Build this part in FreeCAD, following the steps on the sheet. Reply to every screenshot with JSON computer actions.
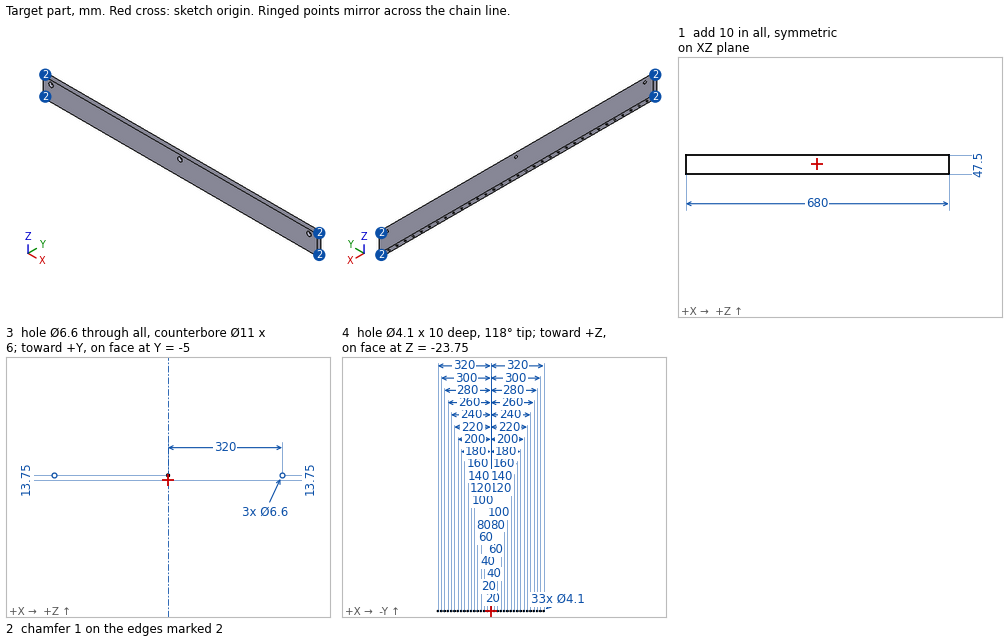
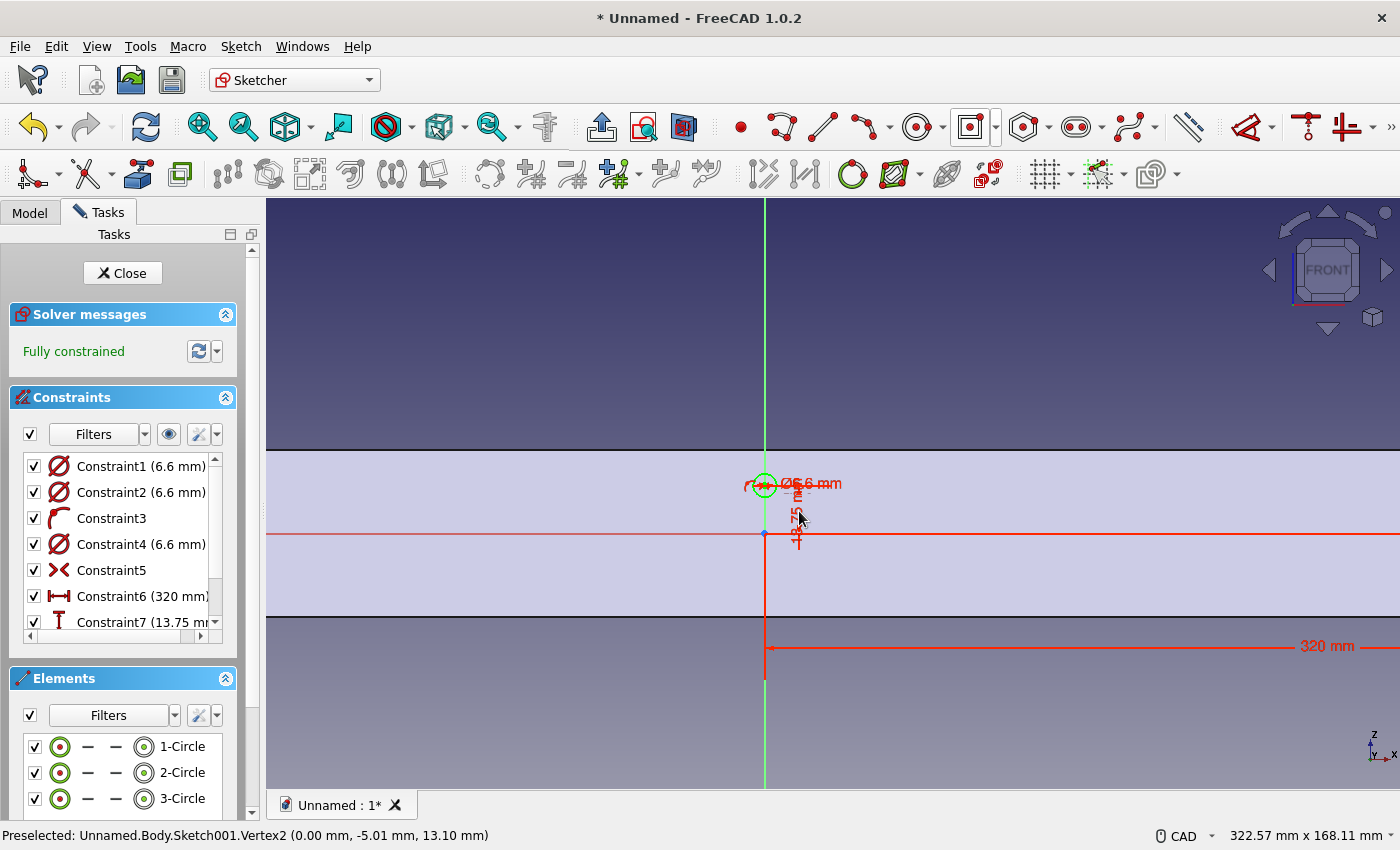
{"action": "left_click", "coordinate": [123, 273]}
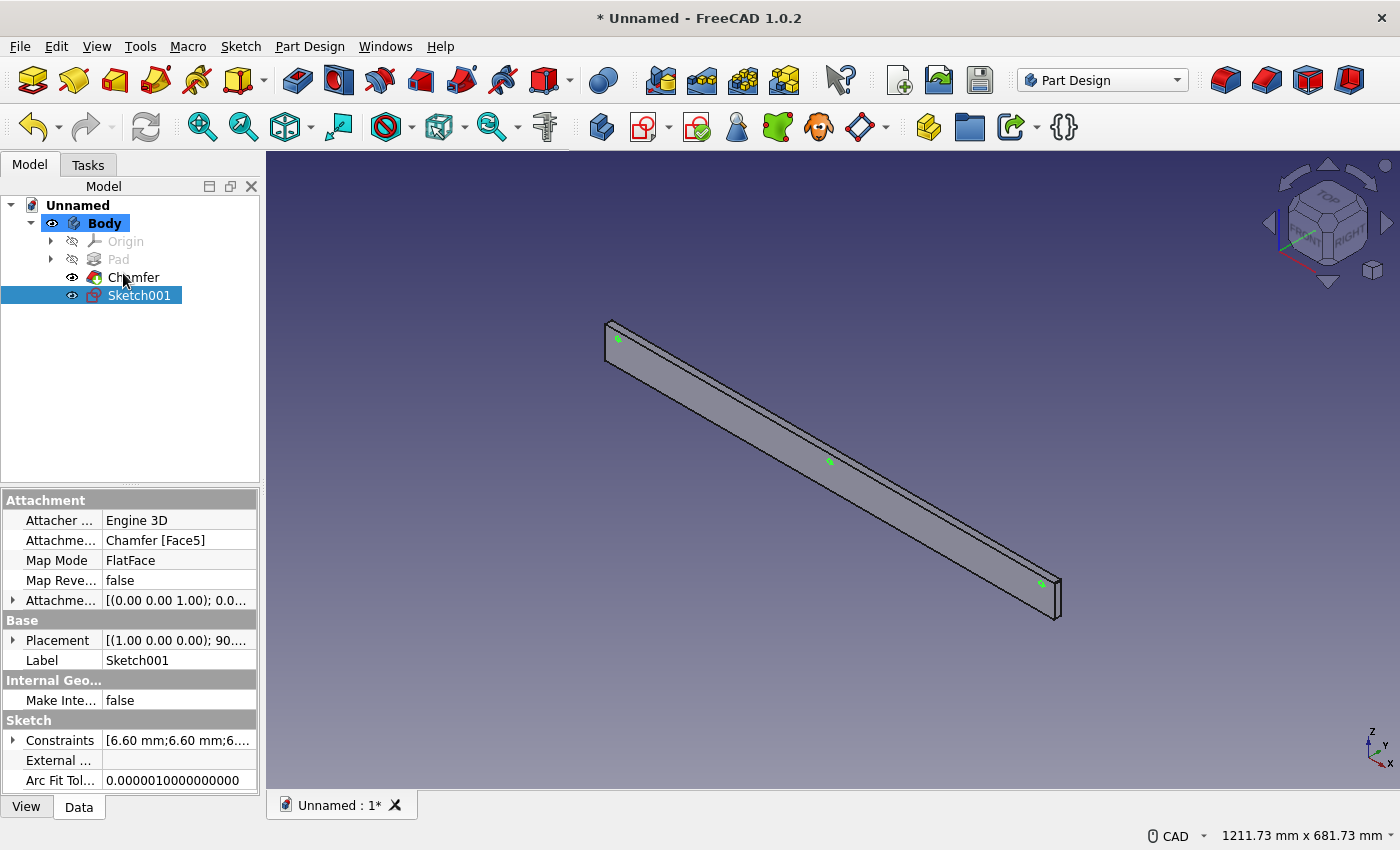
{"action": "left_click", "coordinate": [339, 80]}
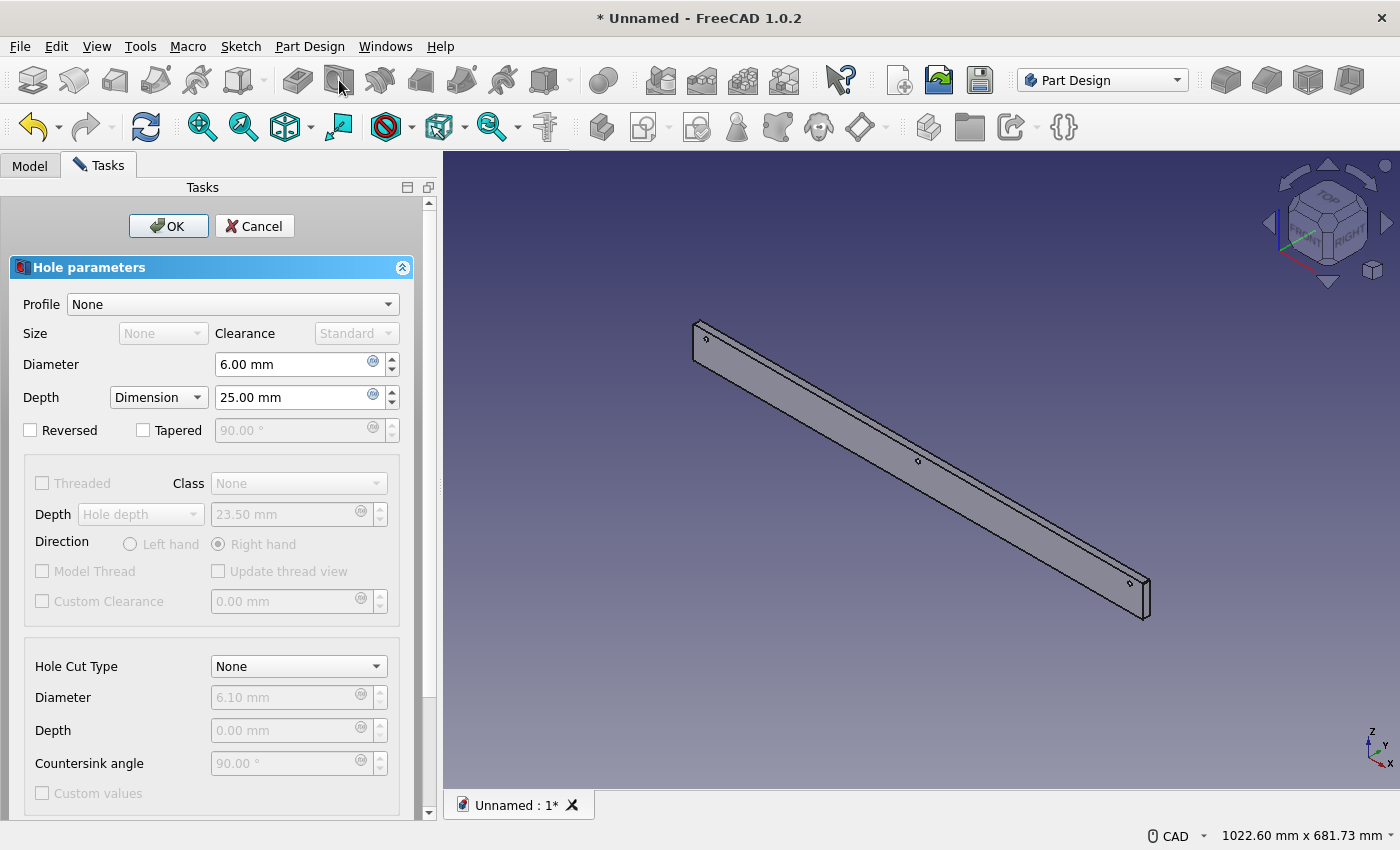
{"action": "triple_click", "coordinate": [300, 364]}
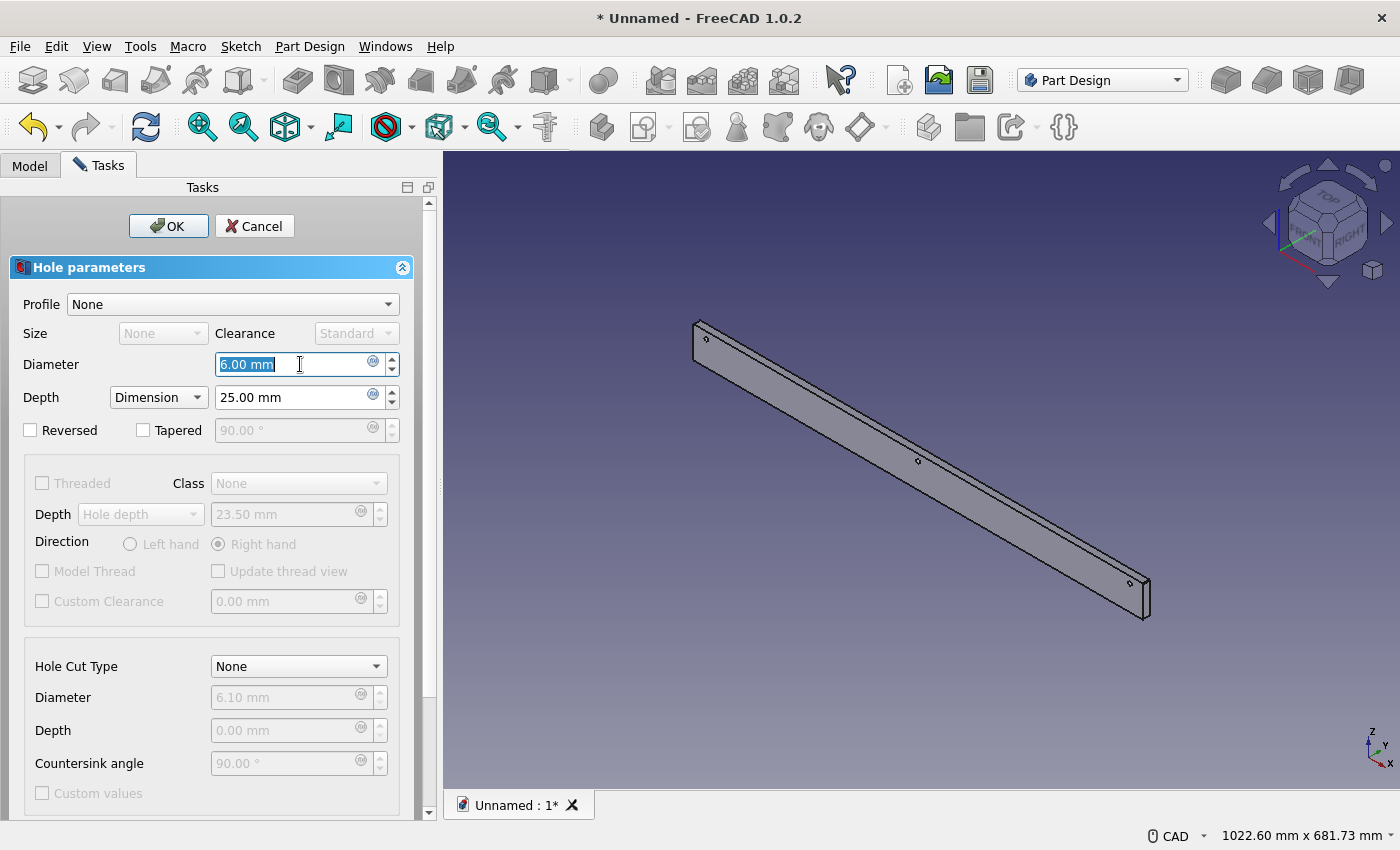
{"action": "type", "text": "6.6"}
{"action": "key", "text": "Tab"}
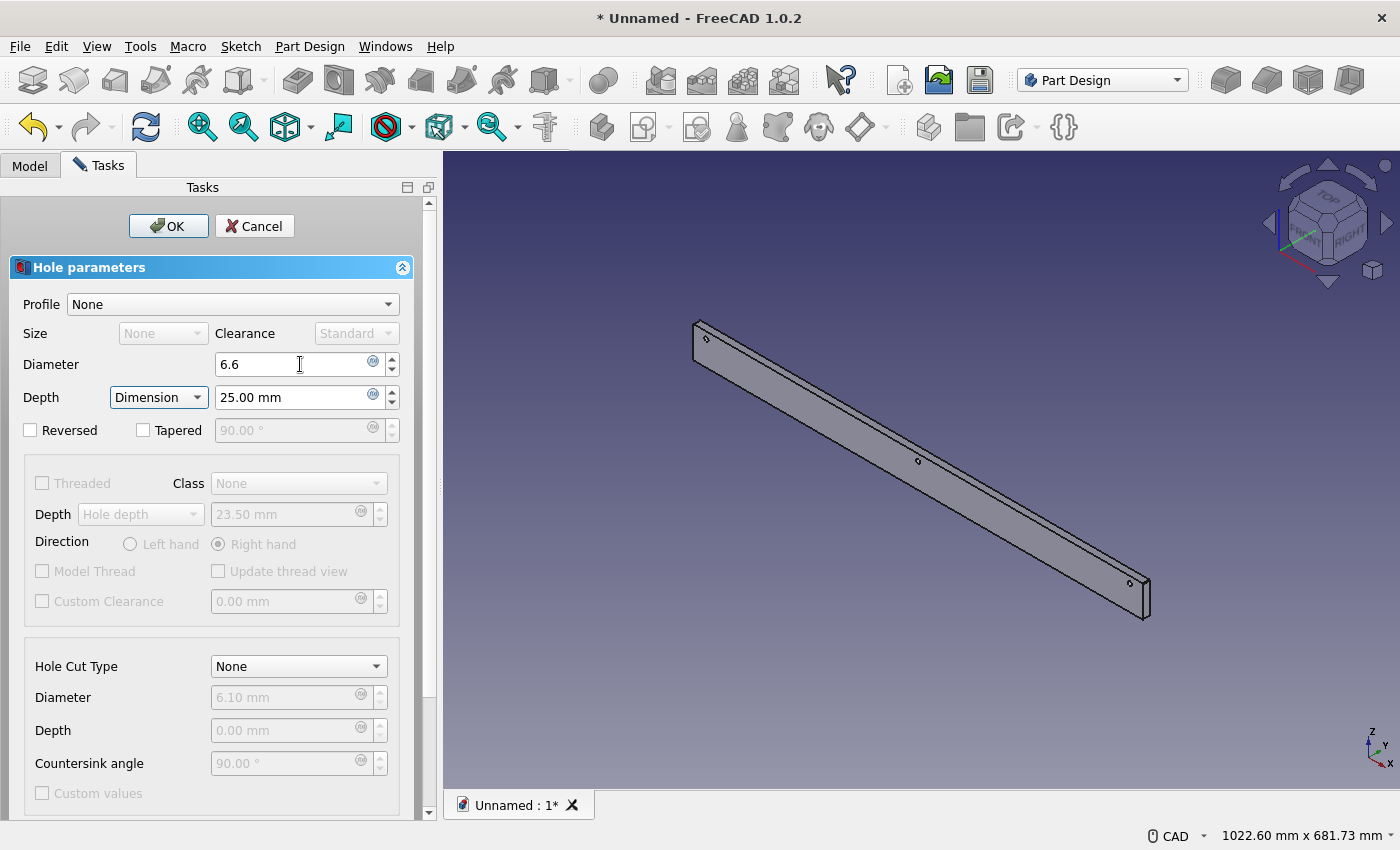
{"action": "left_click", "coordinate": [160, 398]}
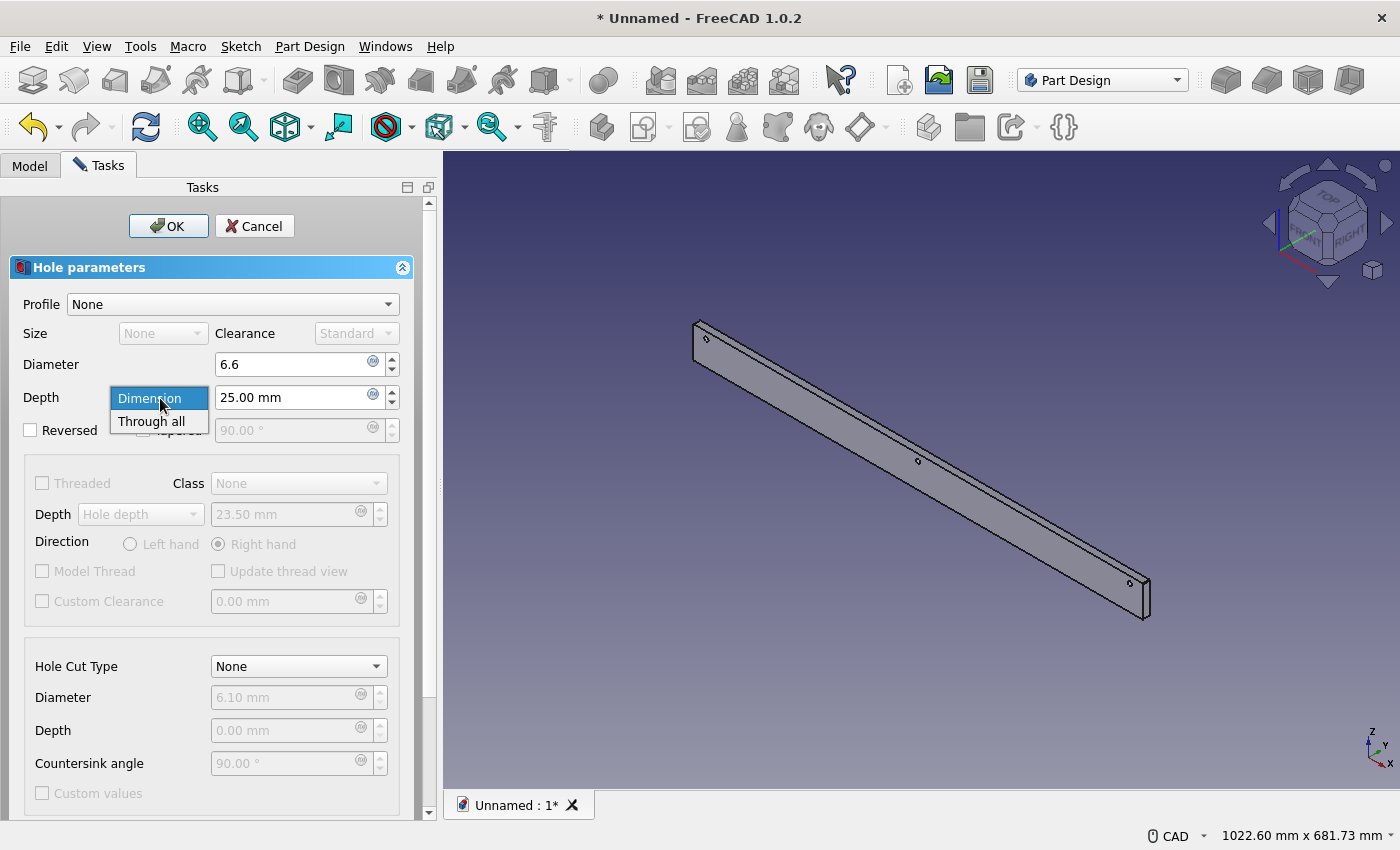
{"action": "left_click", "coordinate": [158, 422]}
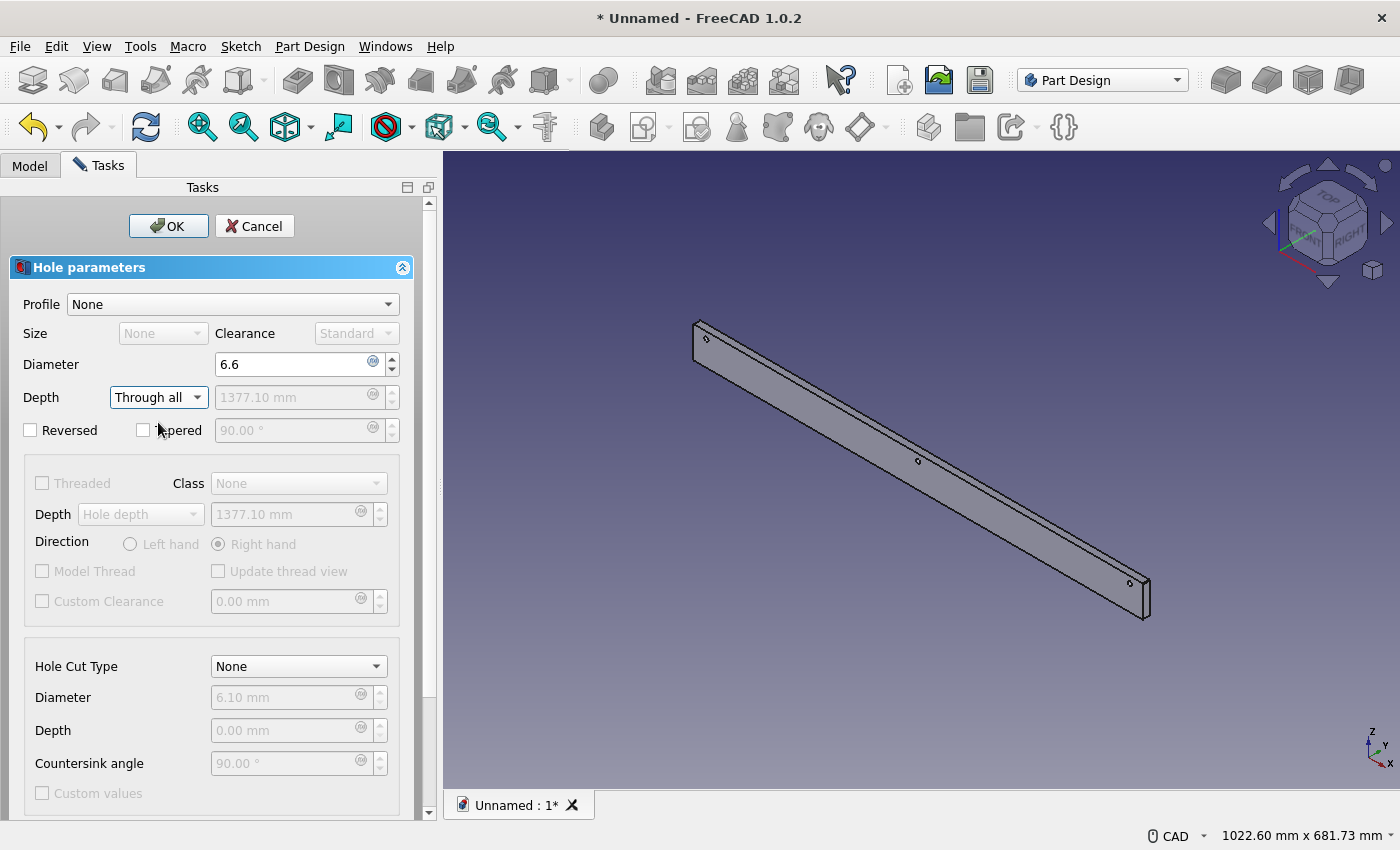
{"action": "left_click", "coordinate": [300, 666]}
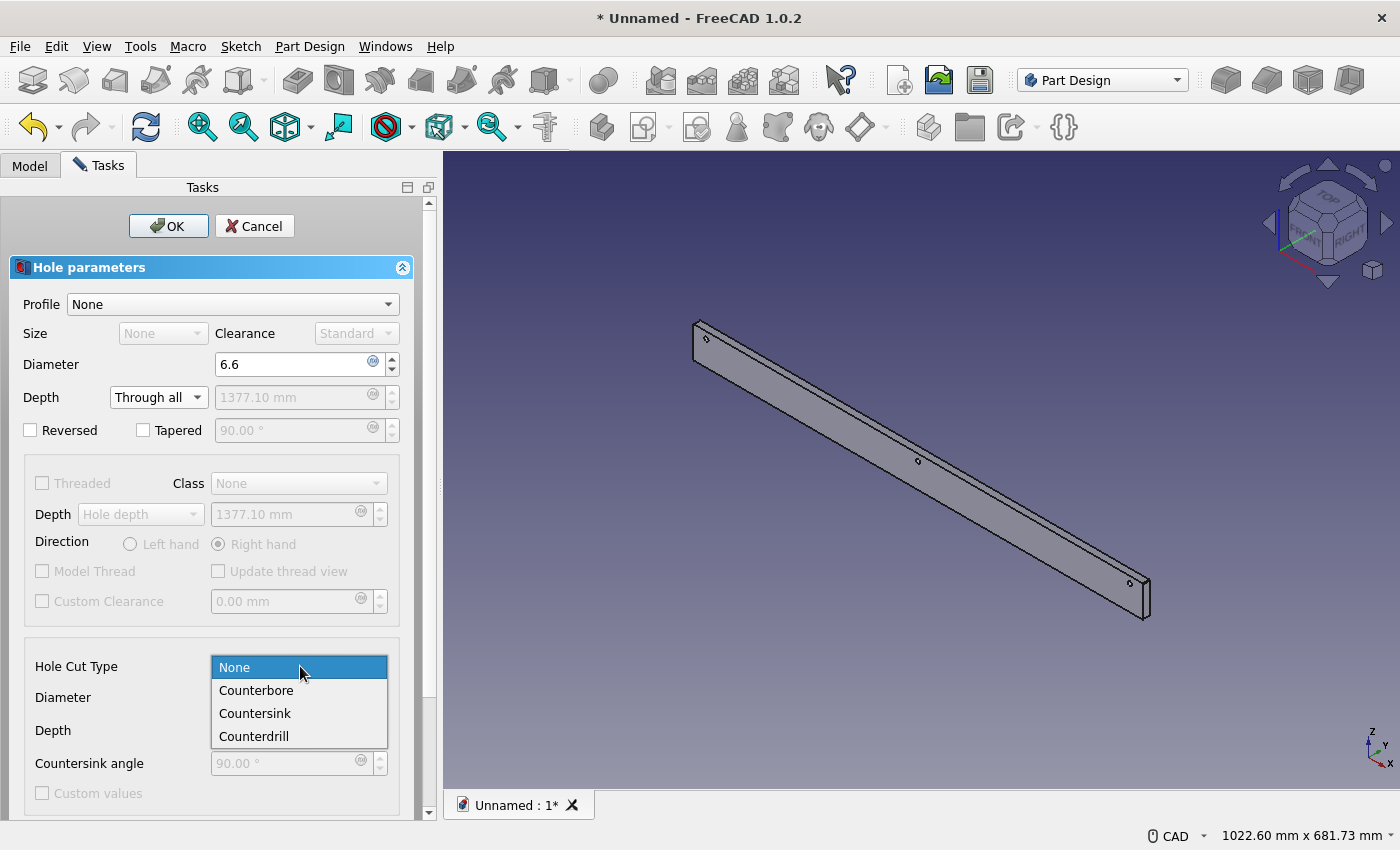
{"action": "left_click", "coordinate": [298, 690]}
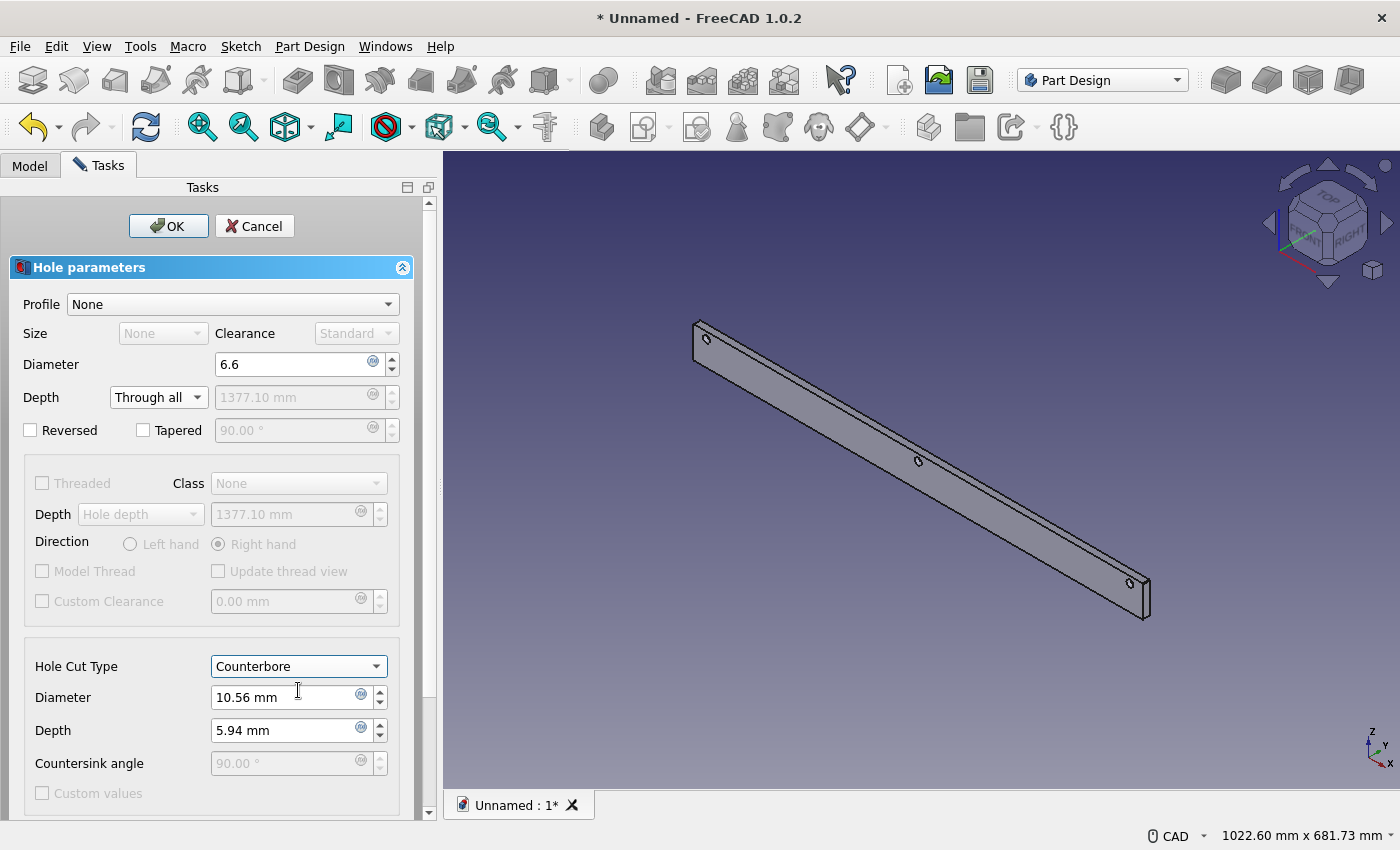
{"action": "triple_click", "coordinate": [292, 698]}